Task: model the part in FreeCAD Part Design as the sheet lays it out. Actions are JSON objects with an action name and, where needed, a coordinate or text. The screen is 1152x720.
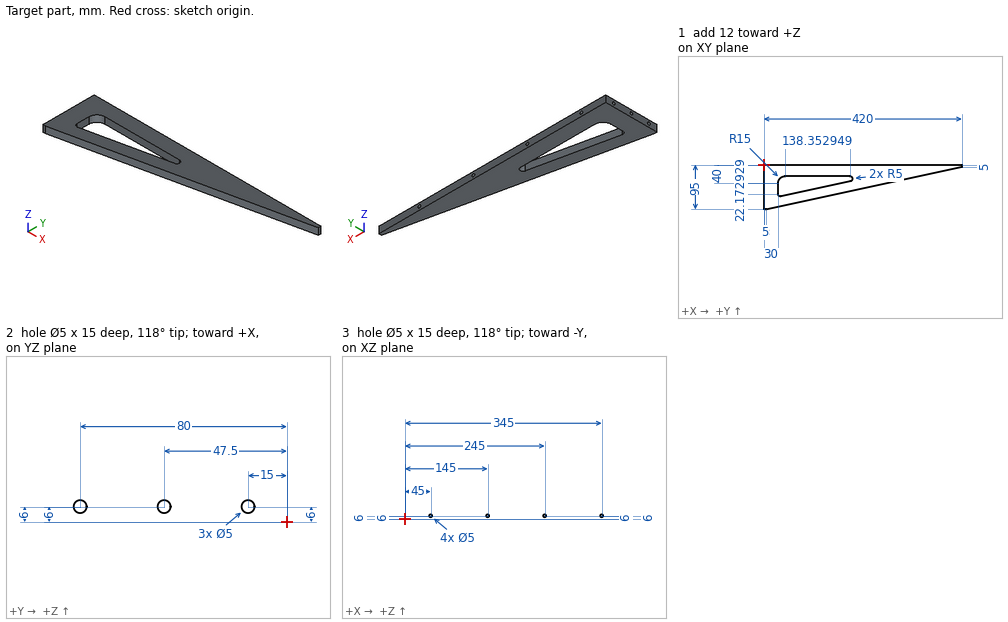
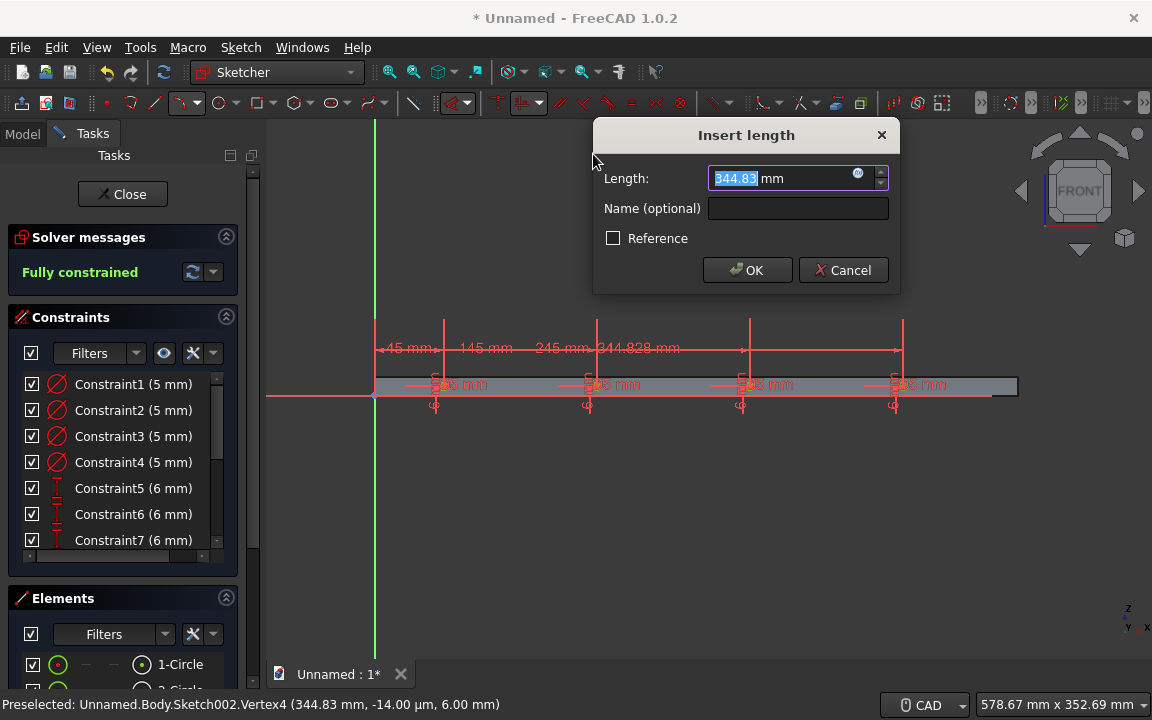
{"action": "type", "text": "345"}
{"action": "key", "text": "Return"}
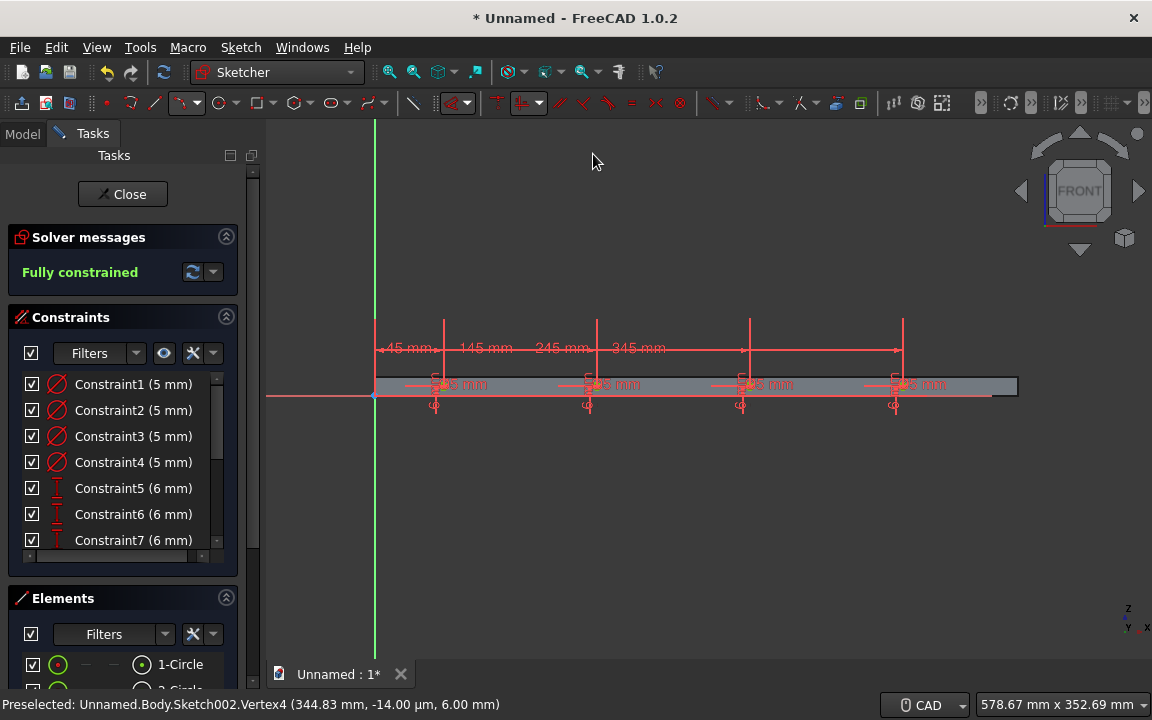
{"action": "left_click", "coordinate": [123, 194]}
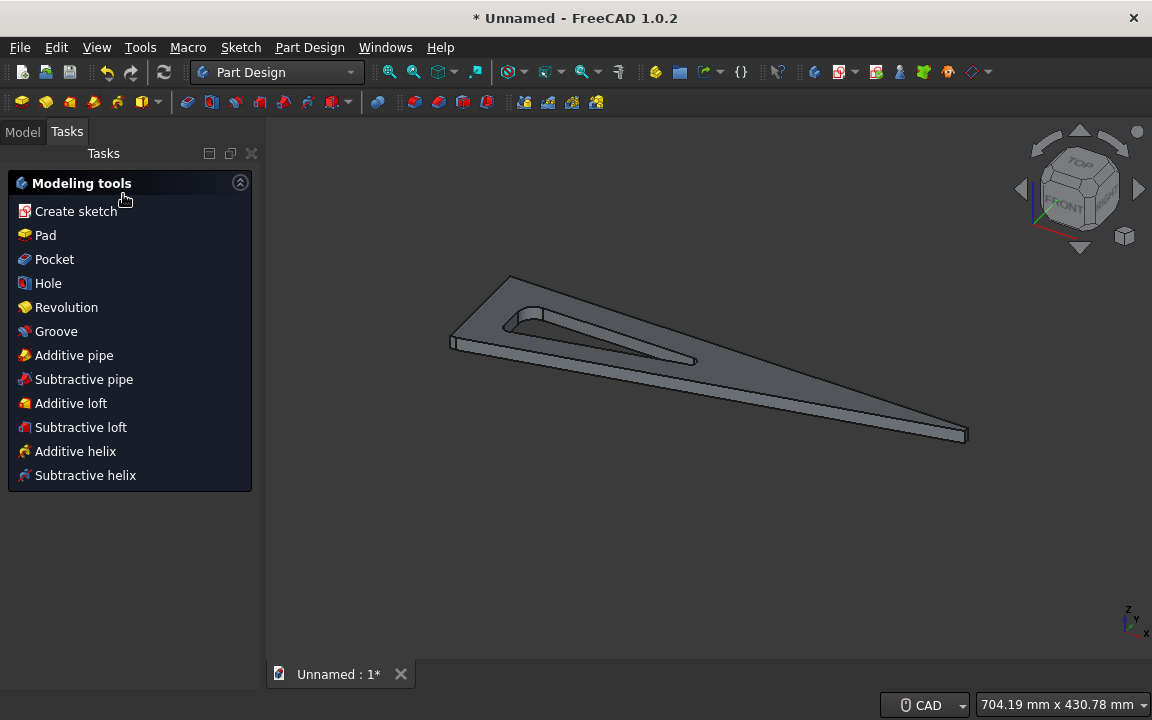
{"action": "left_click", "coordinate": [212, 102]}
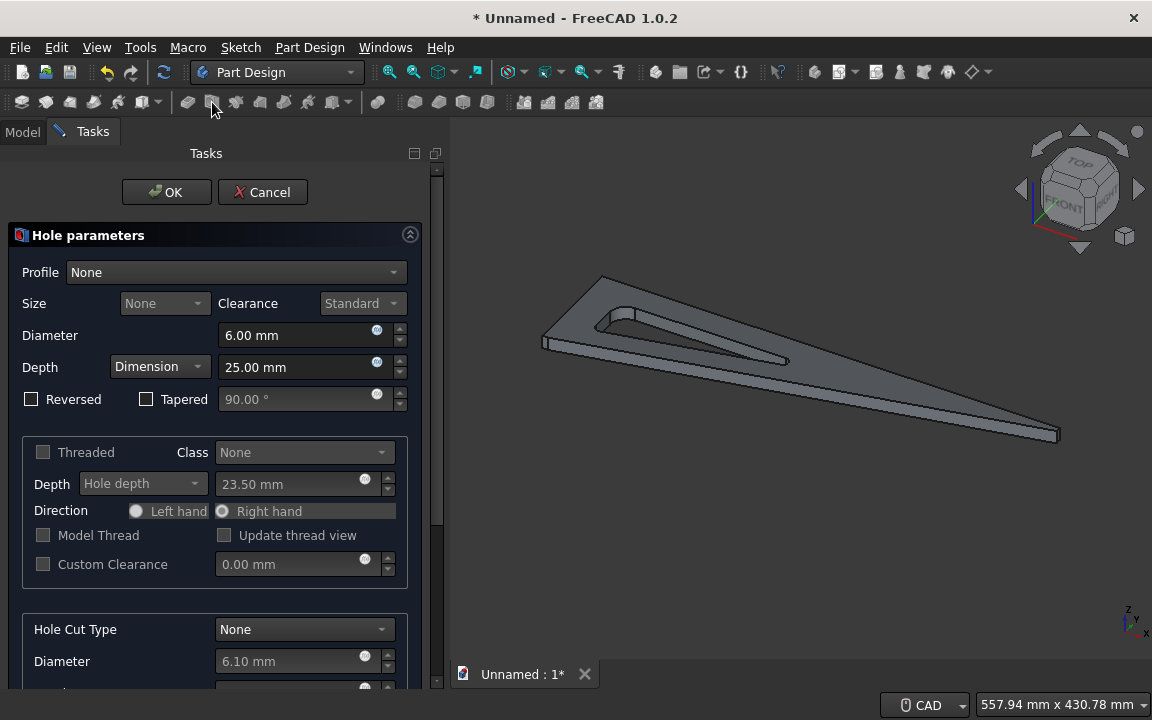
{"action": "triple_click", "coordinate": [305, 335]}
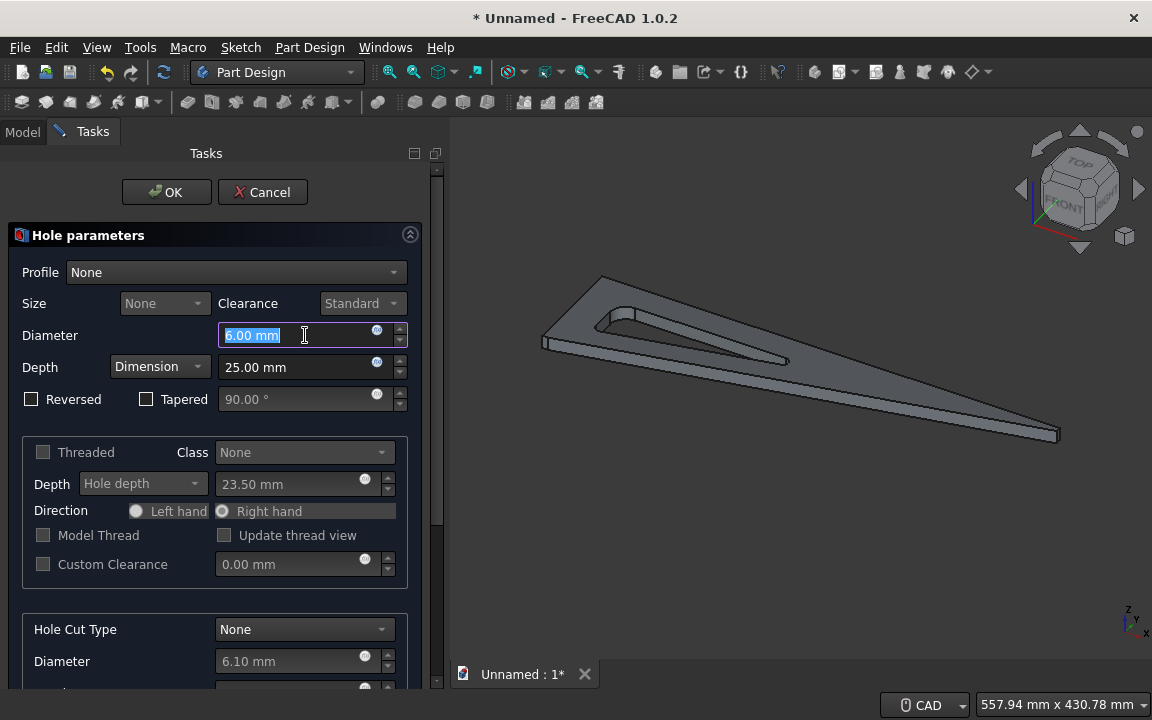
{"action": "type", "text": "5"}
{"action": "key", "text": "Tab"}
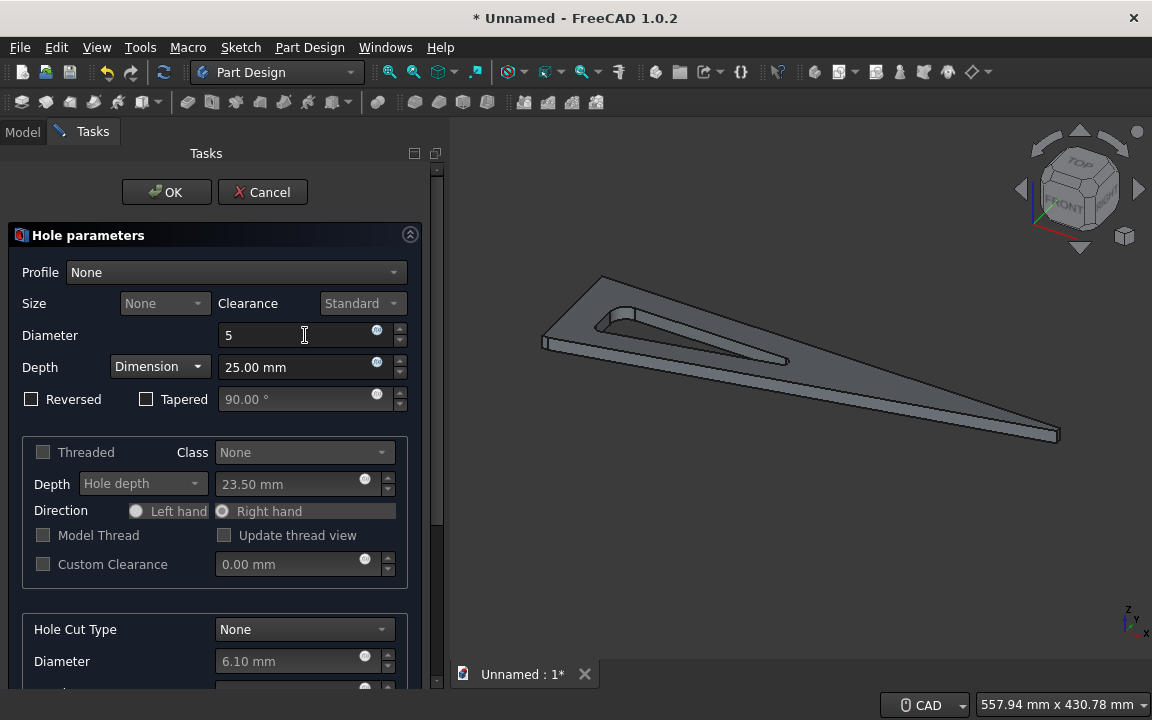
{"action": "triple_click", "coordinate": [305, 367]}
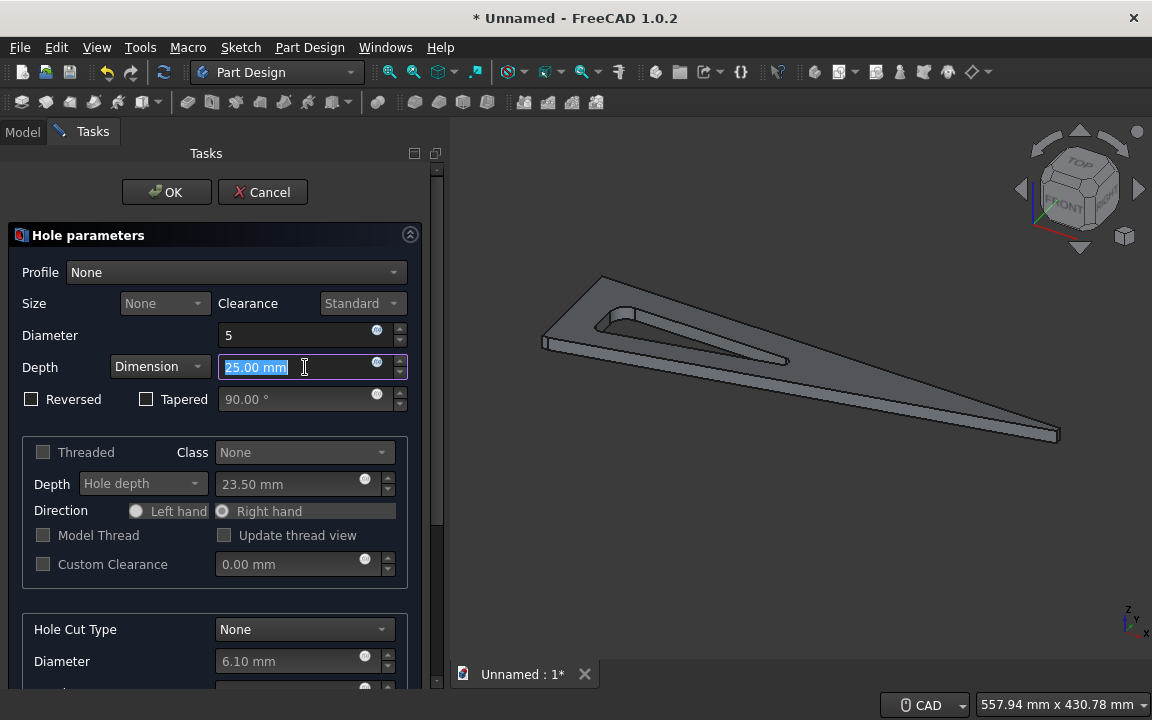
{"action": "type", "text": "15"}
{"action": "key", "text": "Tab"}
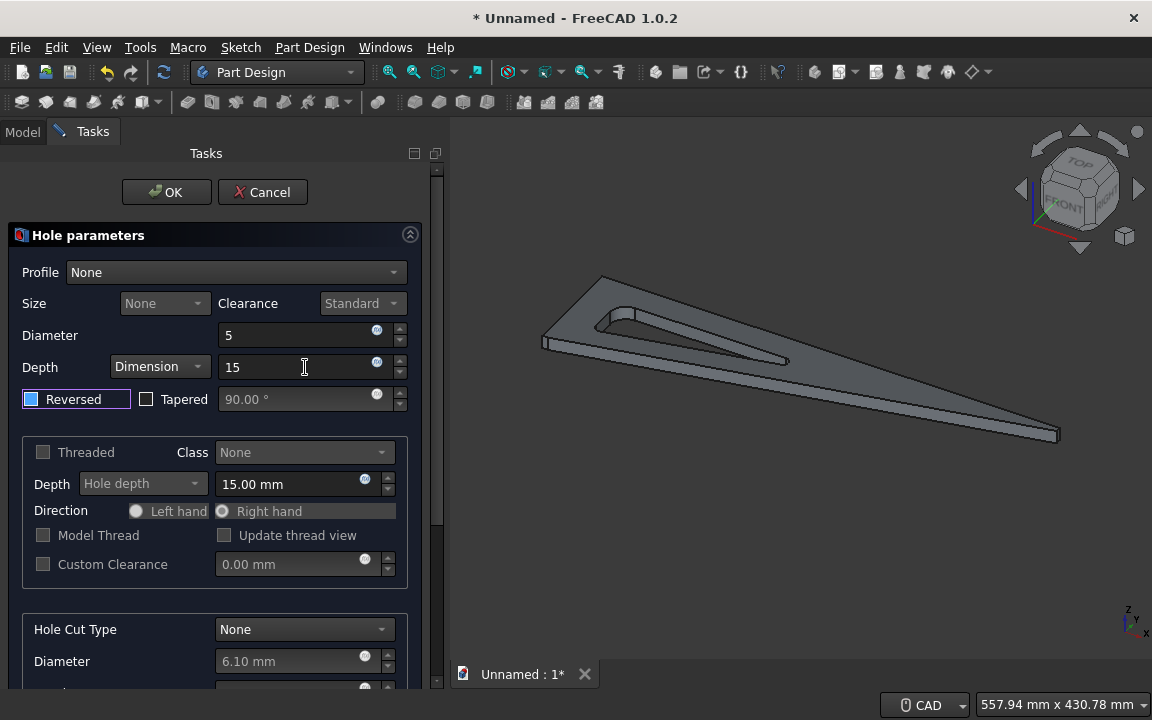
{"action": "left_click", "coordinate": [30, 399]}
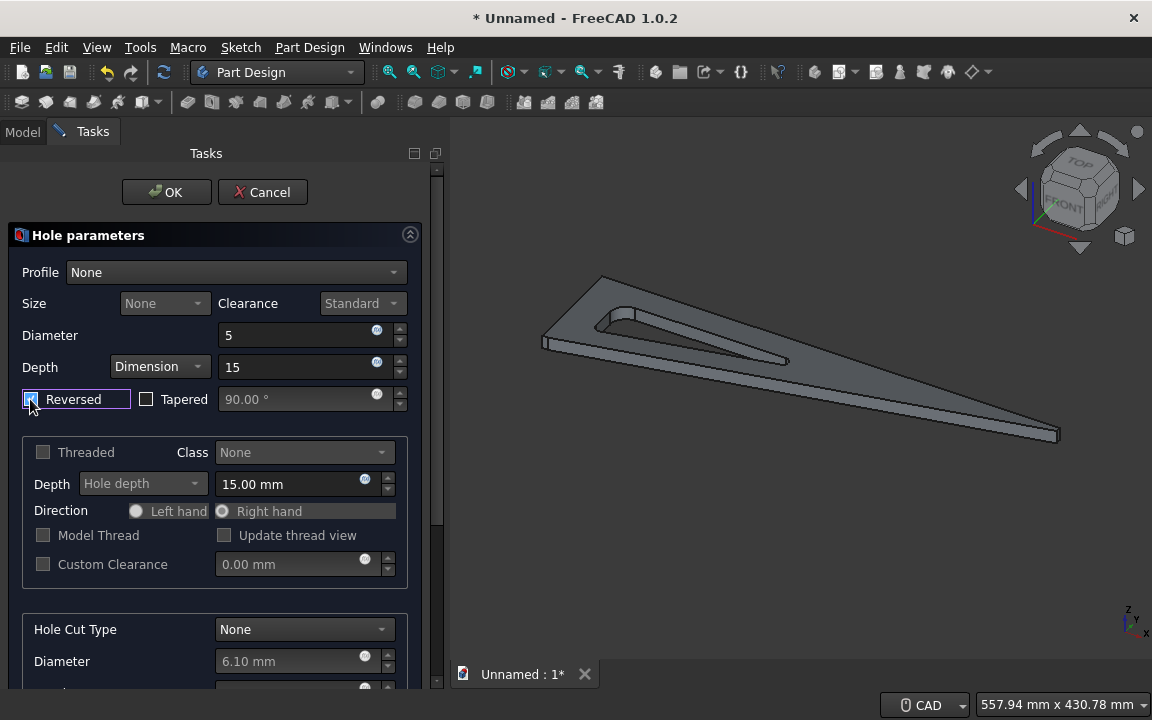
{"action": "left_click", "coordinate": [167, 192]}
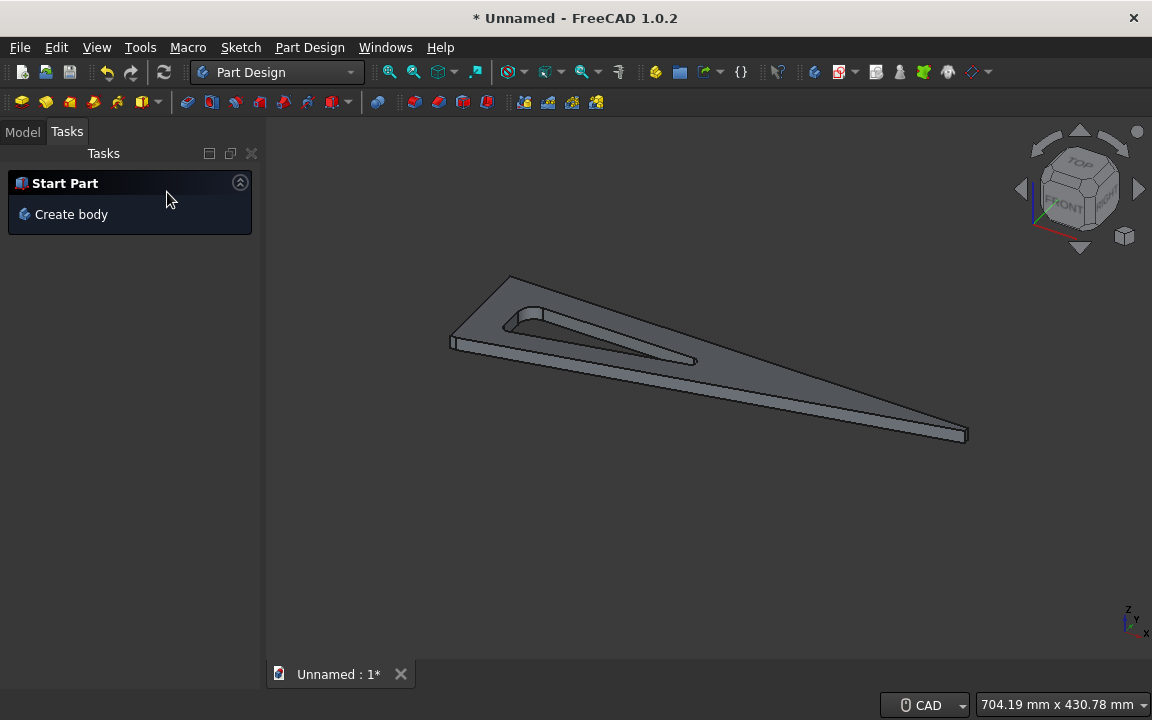
{"action": "key", "text": "0"}